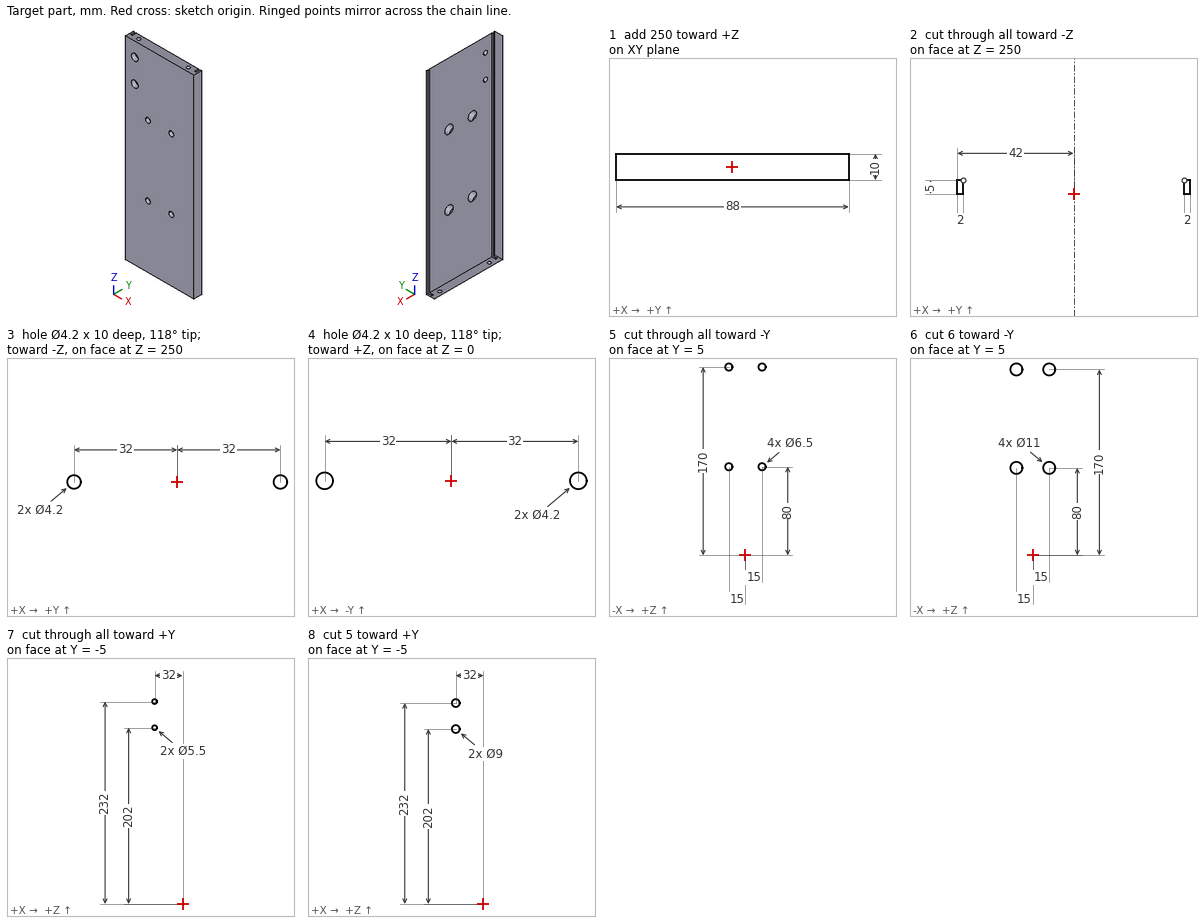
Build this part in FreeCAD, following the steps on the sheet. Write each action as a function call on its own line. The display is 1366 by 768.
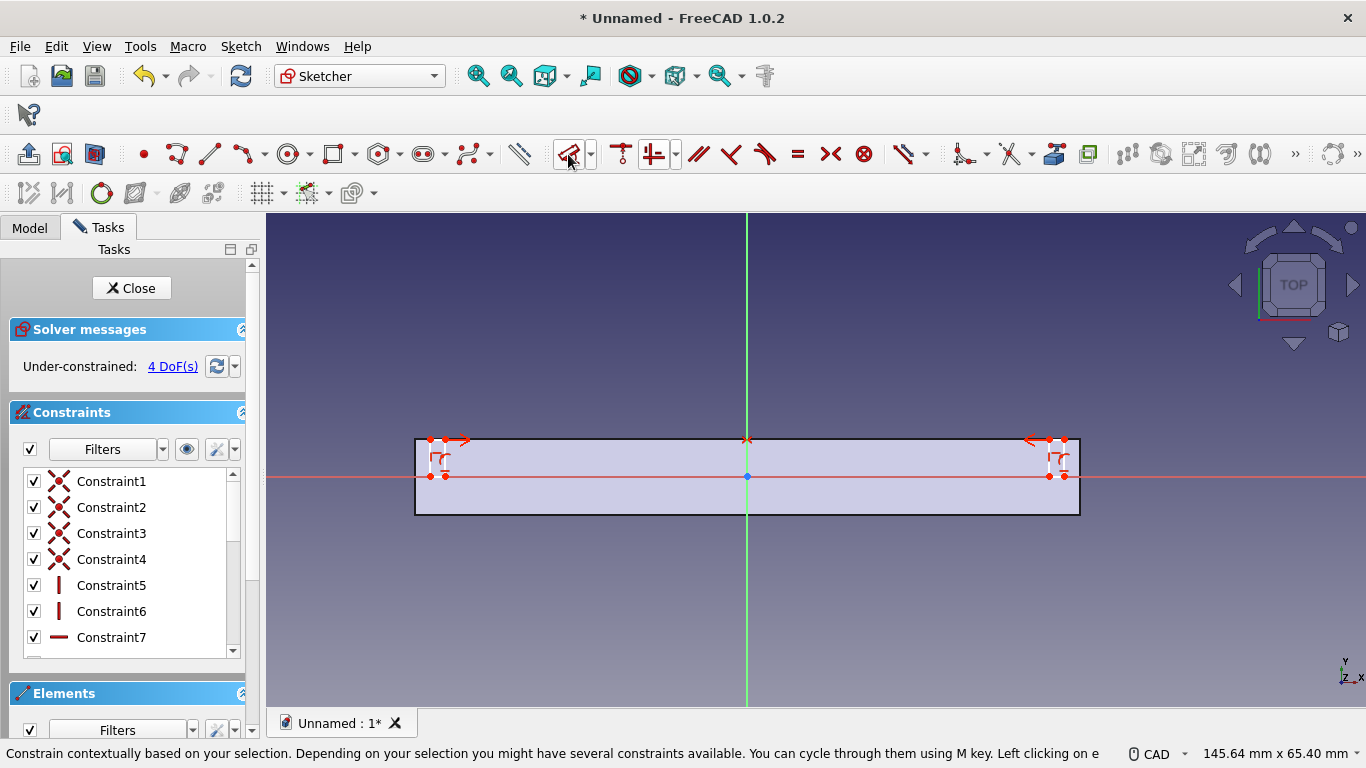
scroll(430, 451, up, 2)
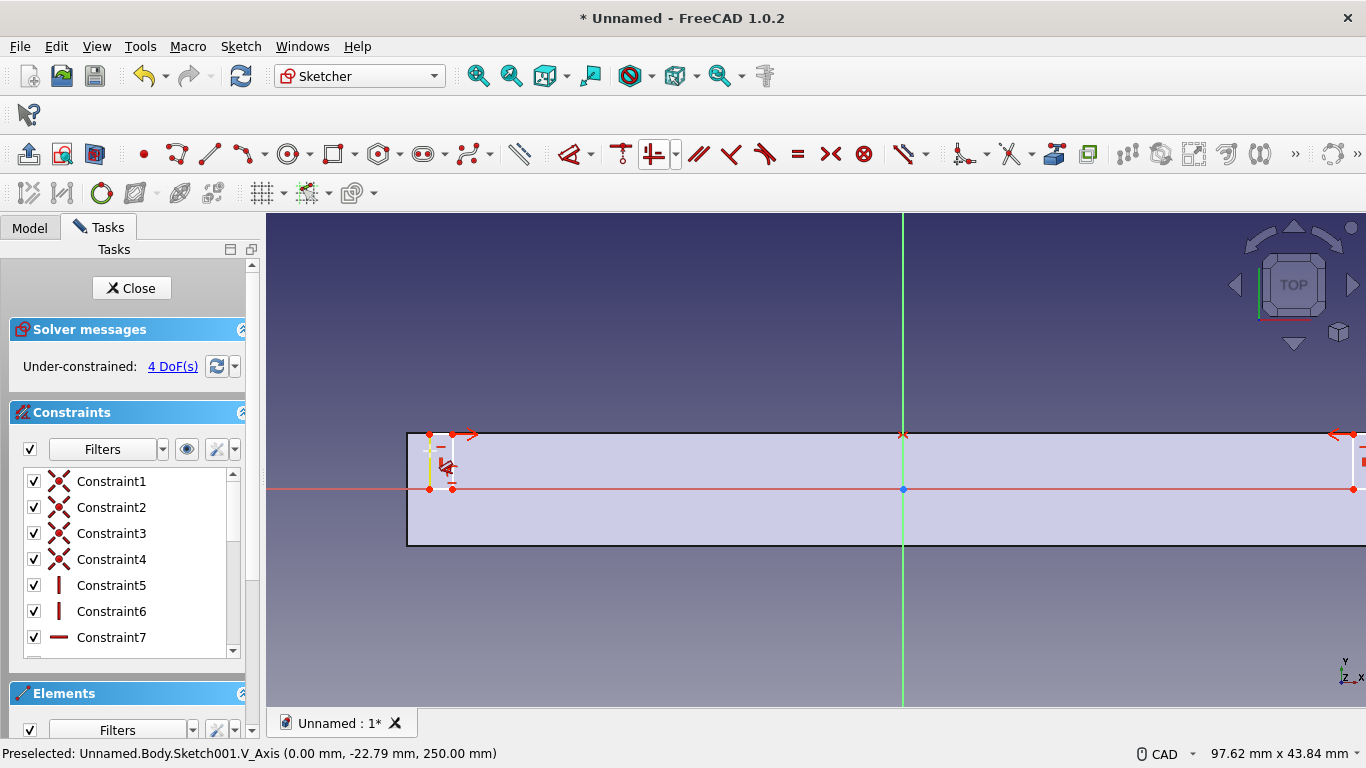
click(430, 451)
click(396, 462)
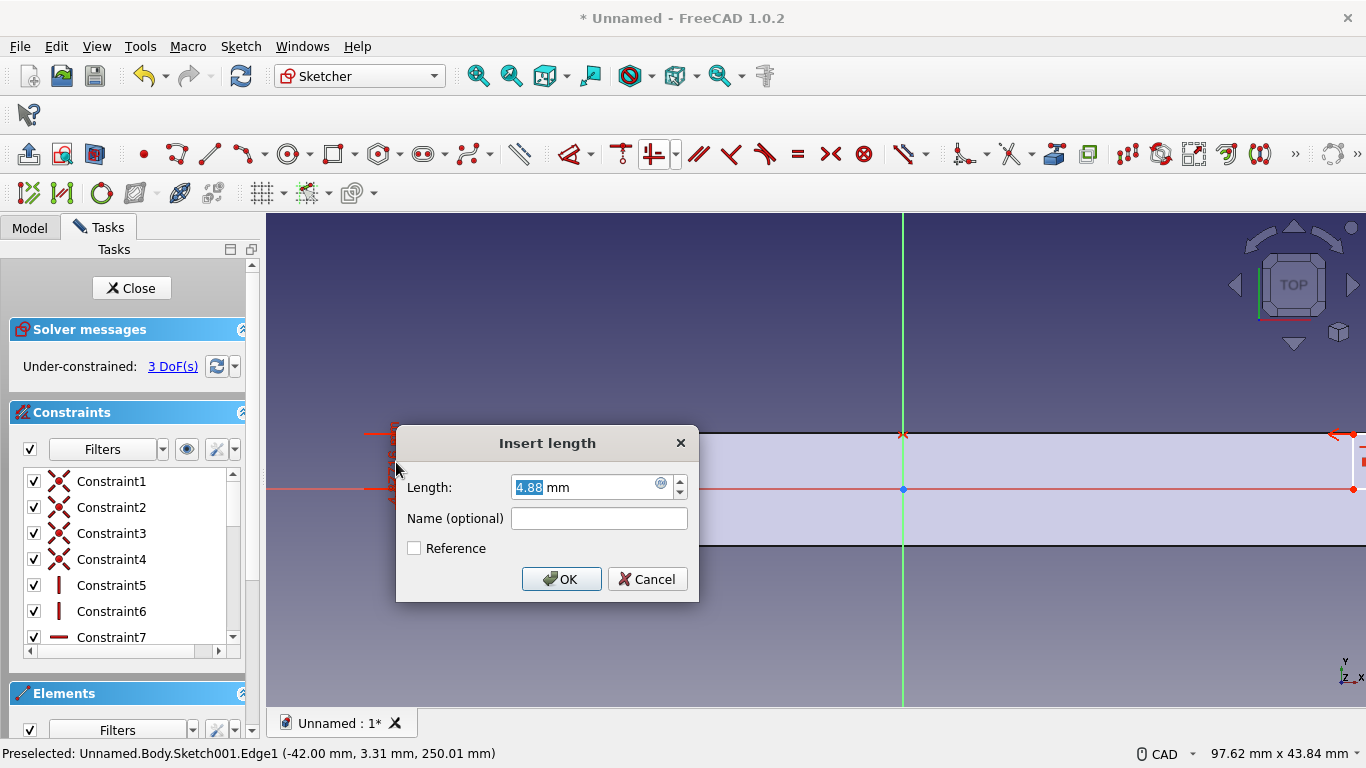
text(5)
key(Return)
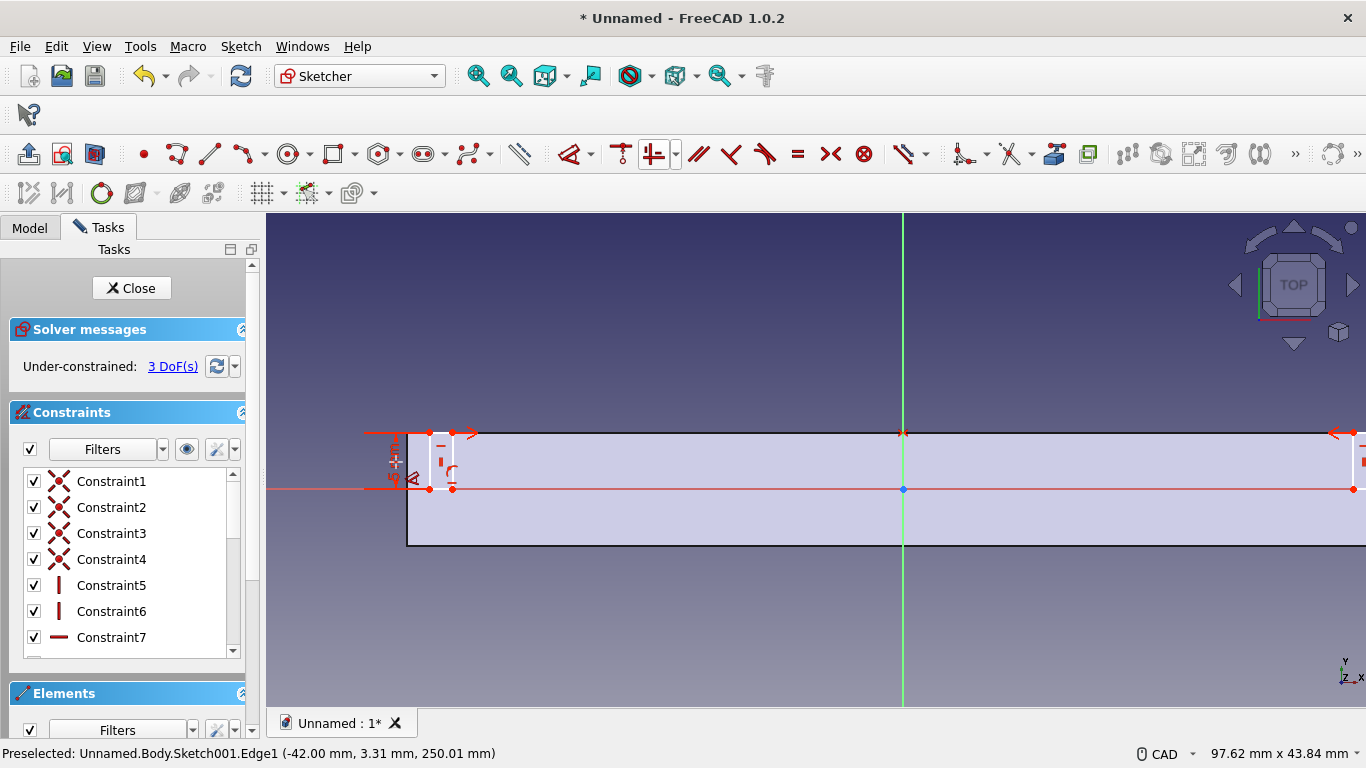
scroll(439, 489, up, 3)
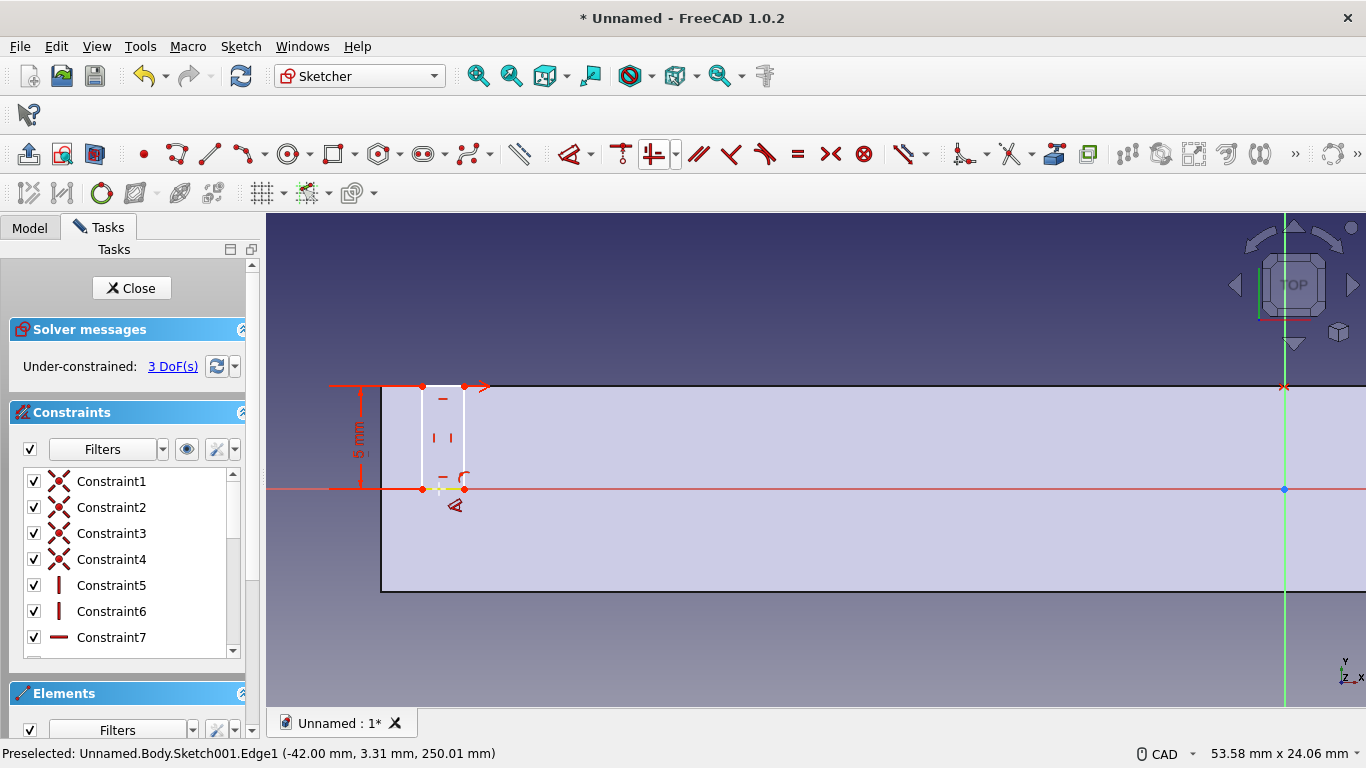
click(439, 489)
click(443, 523)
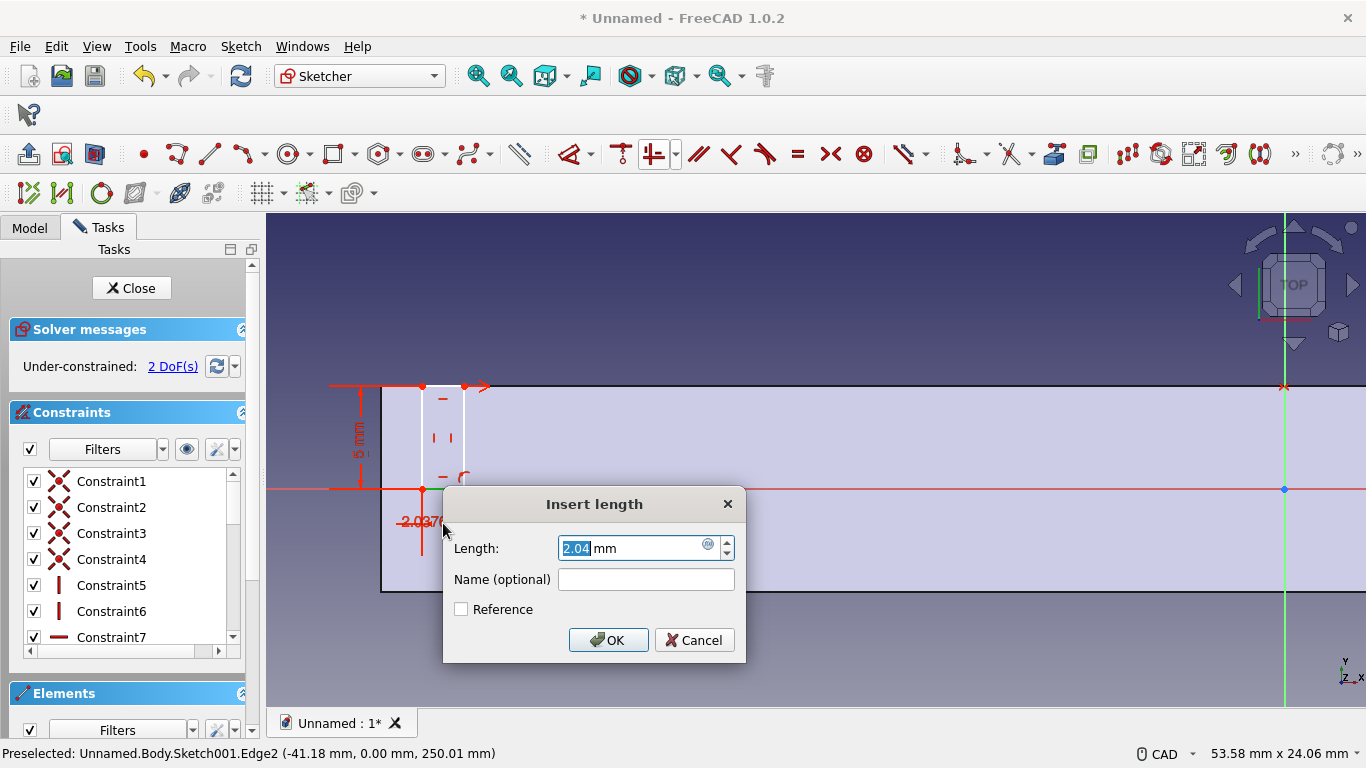
text(2)
key(Return)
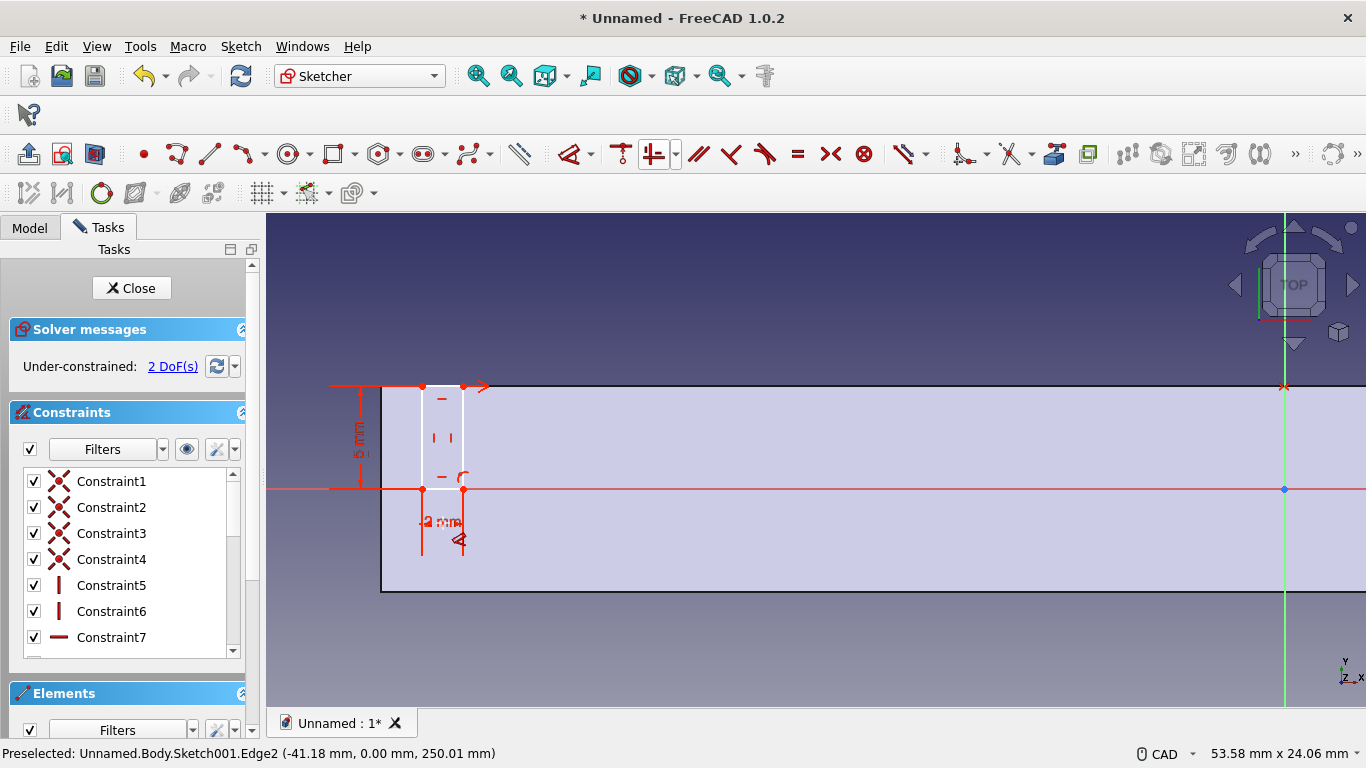
scroll(435, 473, down, 5)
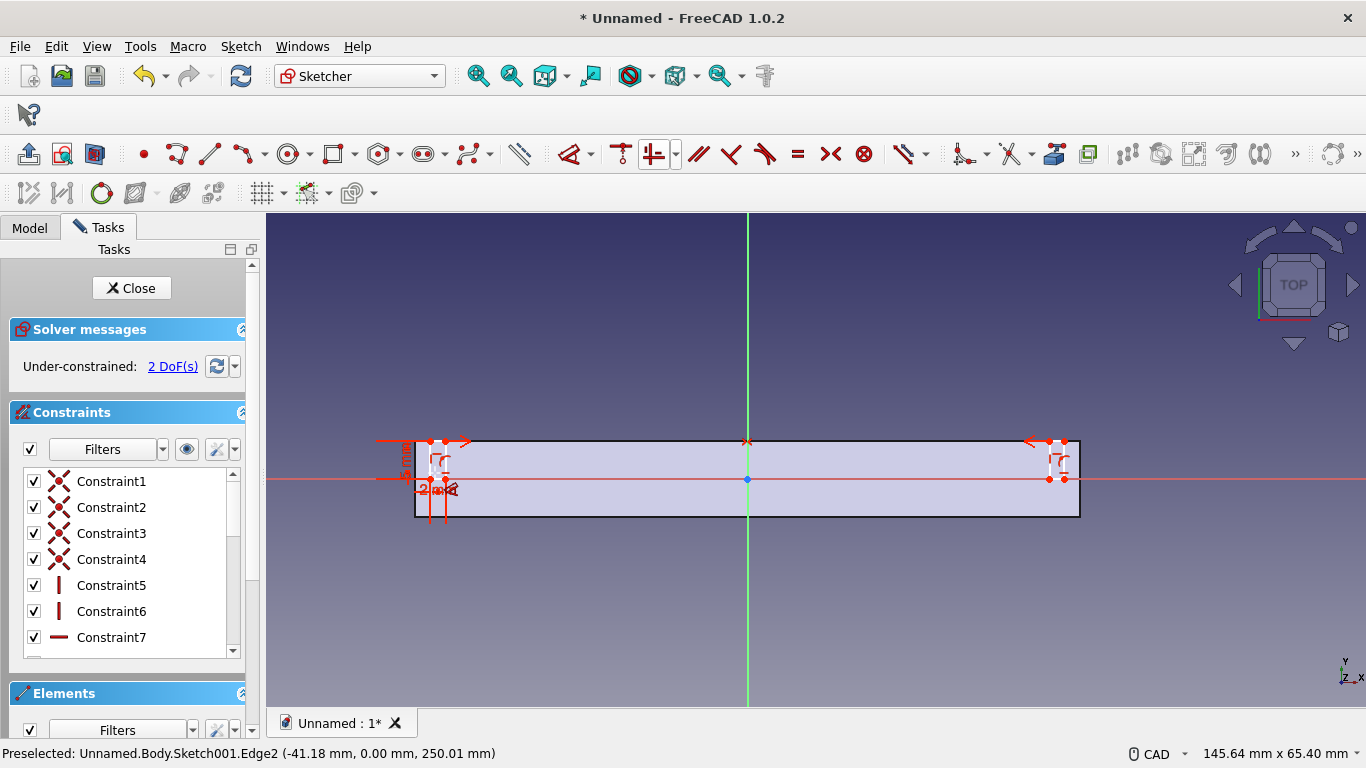
scroll(1054, 479, up, 6)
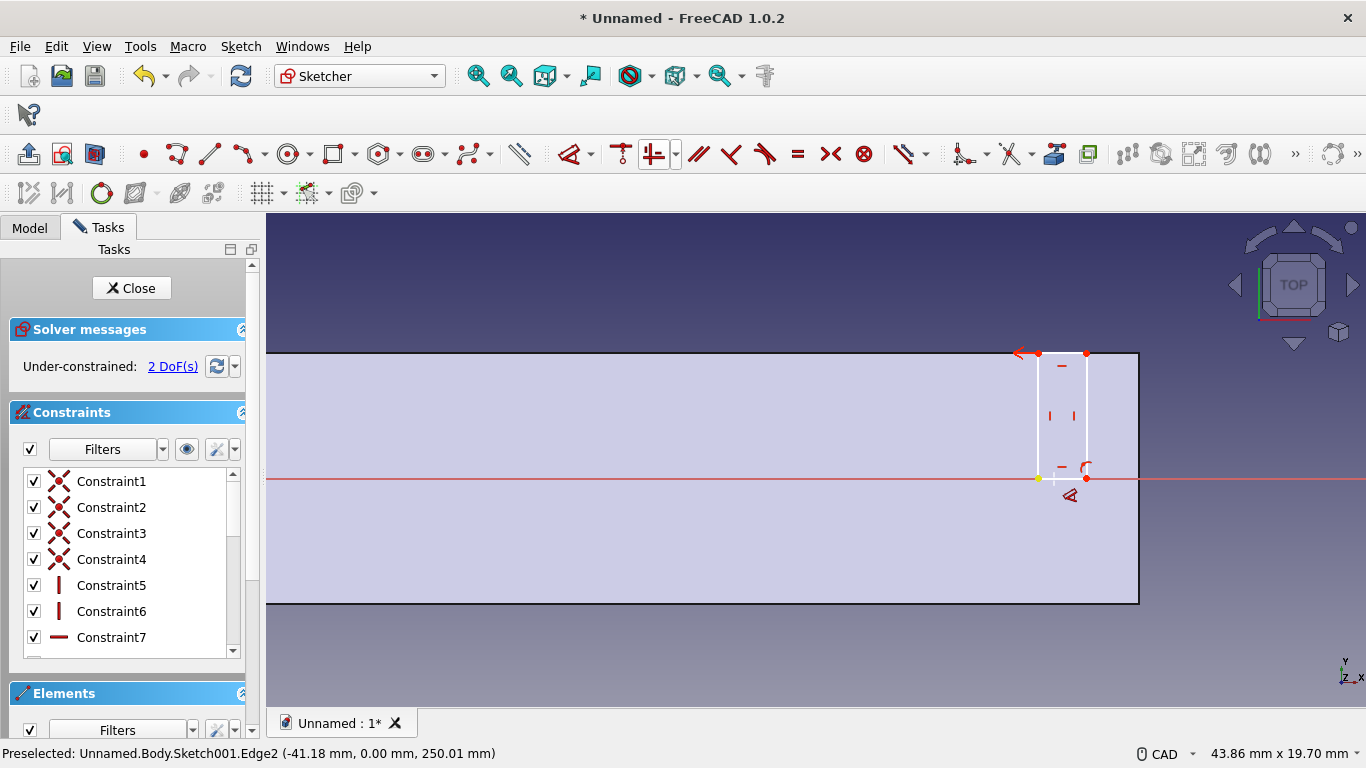
click(1053, 479)
click(1063, 513)